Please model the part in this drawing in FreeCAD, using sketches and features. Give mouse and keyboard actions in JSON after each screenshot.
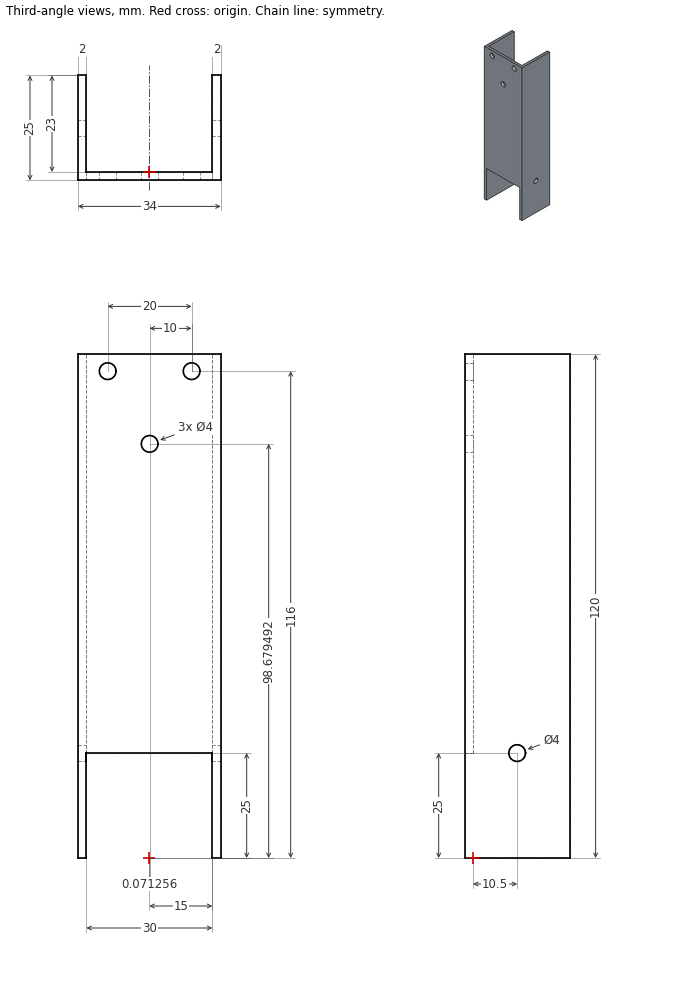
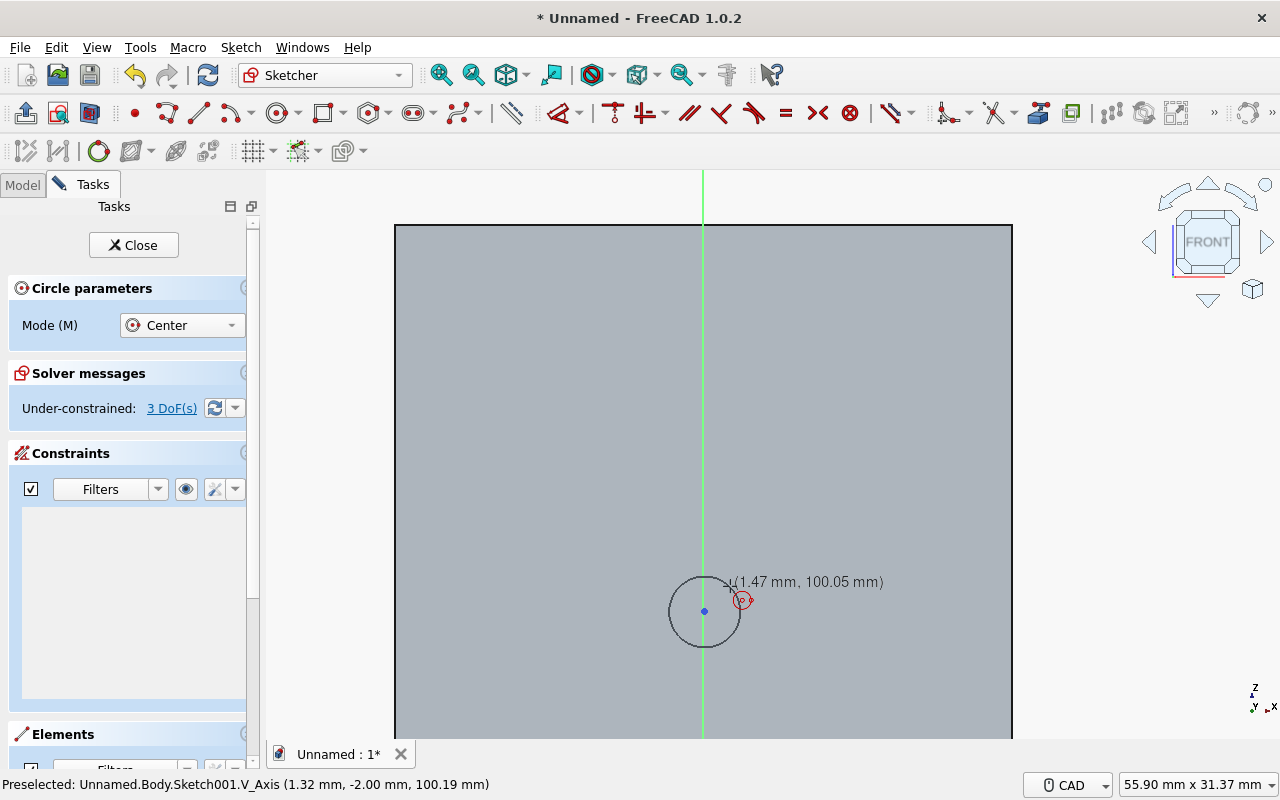
{"action": "left_click", "coordinate": [886, 298]}
{"action": "left_click", "coordinate": [912, 272]}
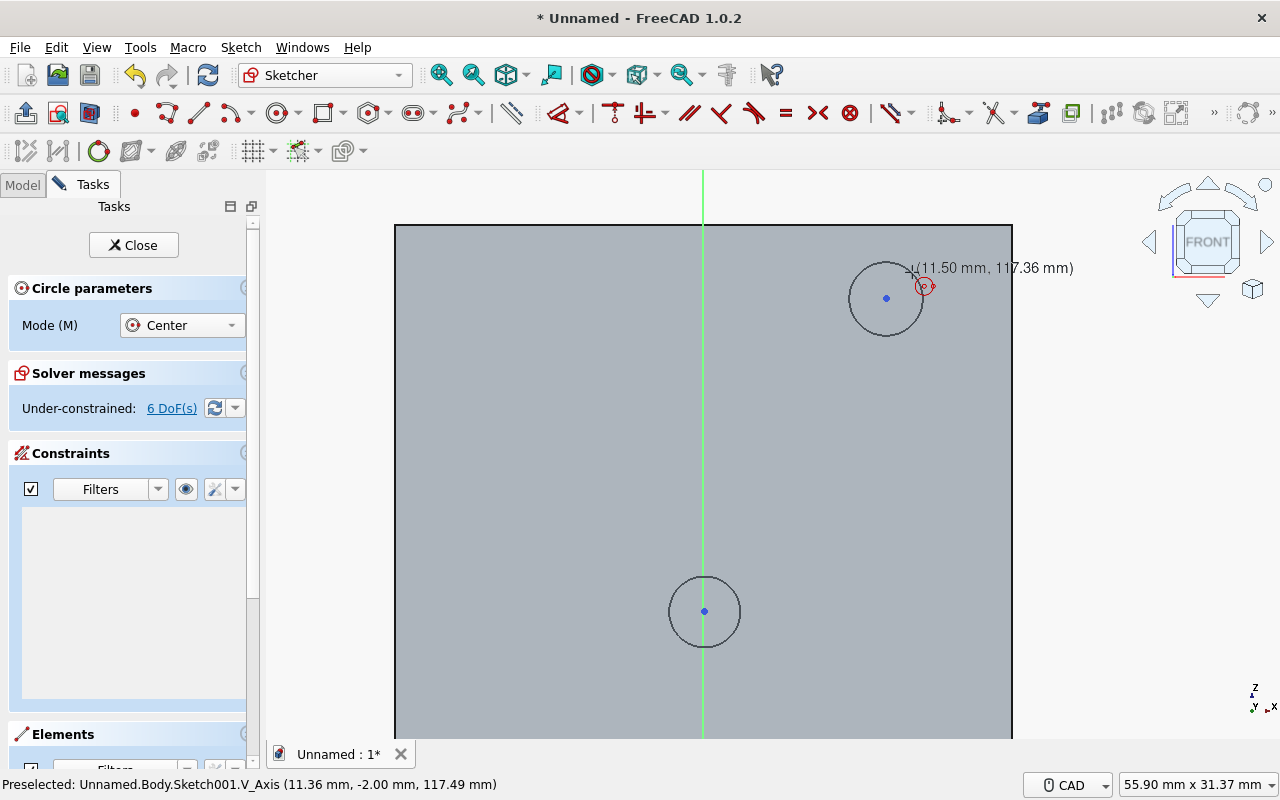
{"action": "left_click", "coordinate": [523, 298]}
{"action": "left_click", "coordinate": [549, 272]}
{"action": "key", "text": "Escape"}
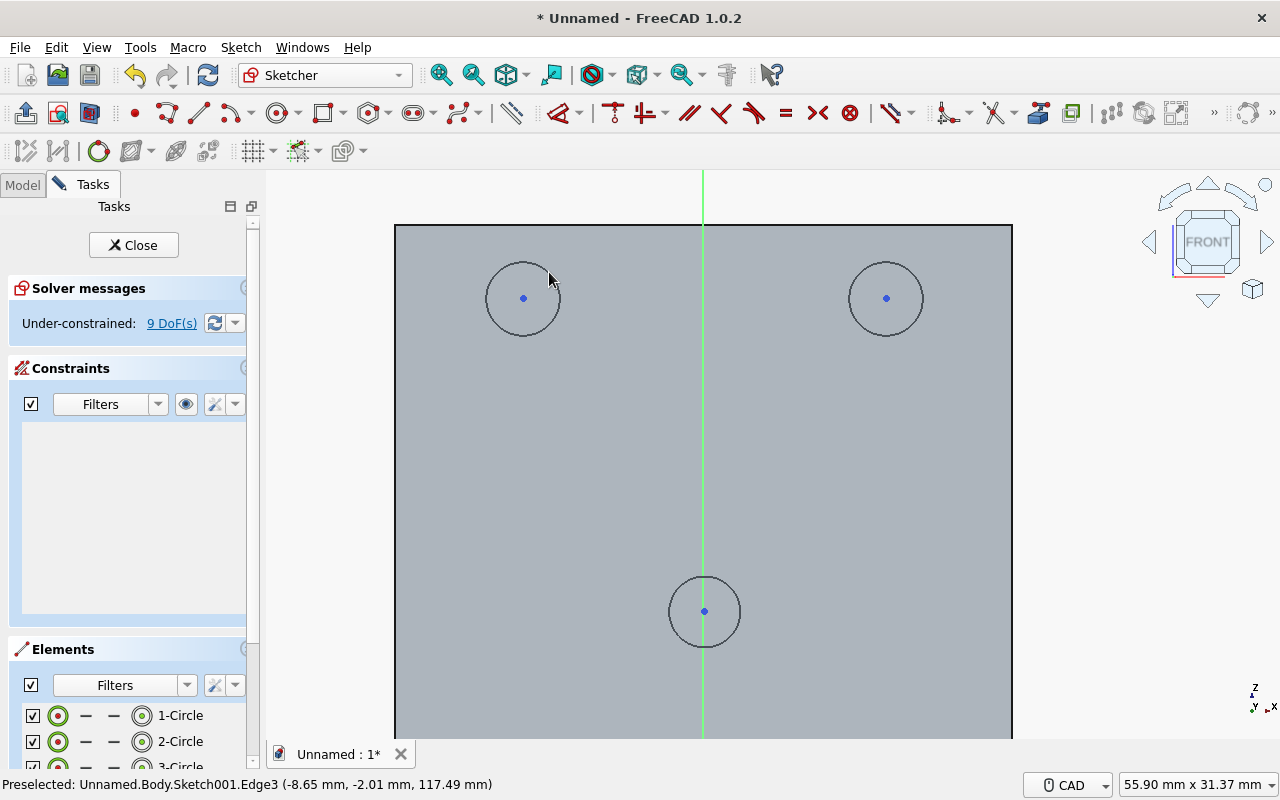
{"action": "left_click", "coordinate": [730, 587]}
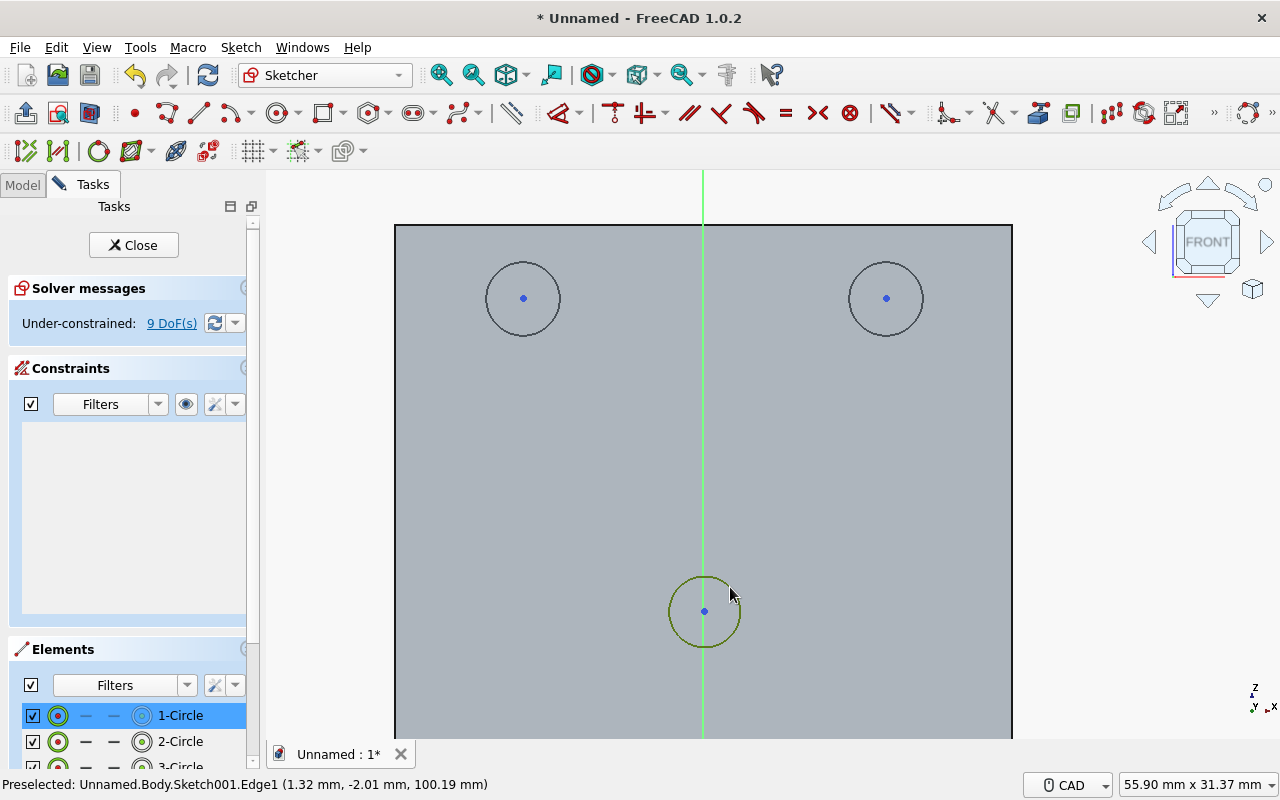
{"action": "left_click", "coordinate": [912, 273]}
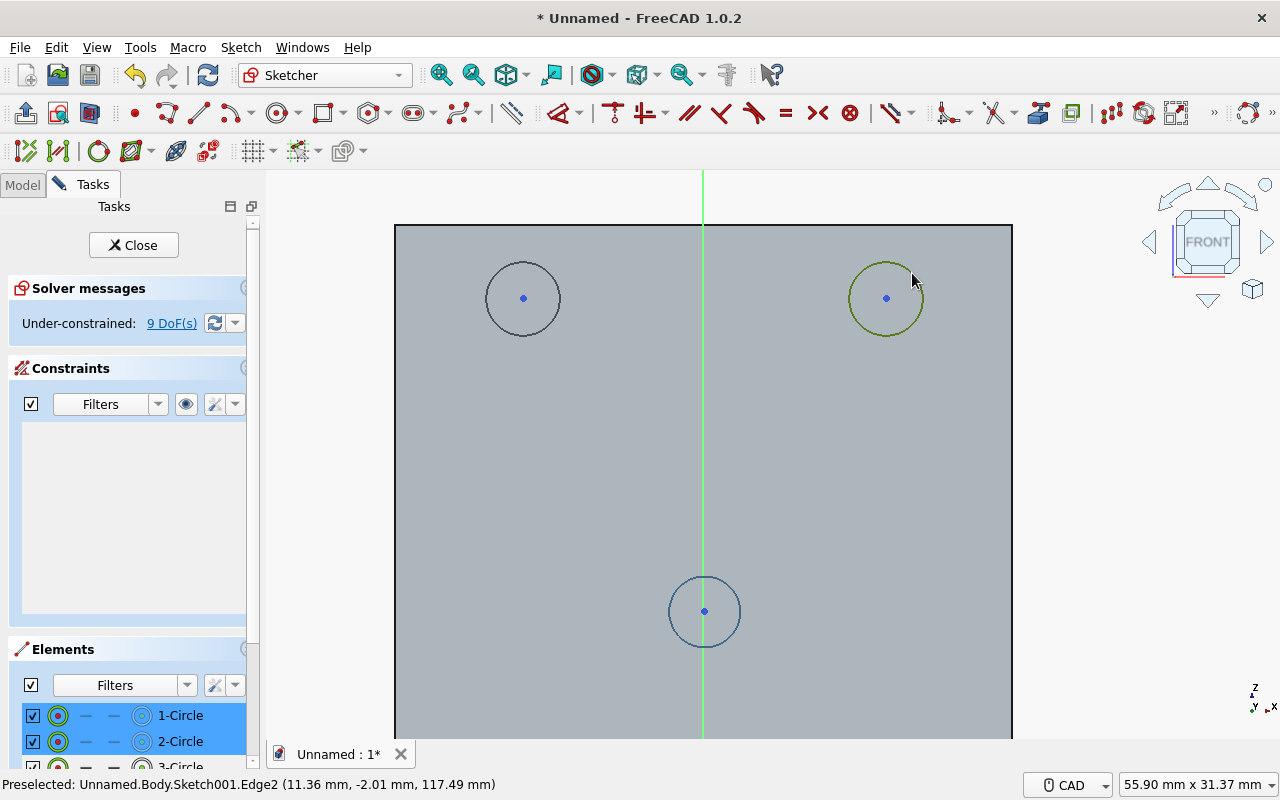
{"action": "left_click", "coordinate": [549, 273]}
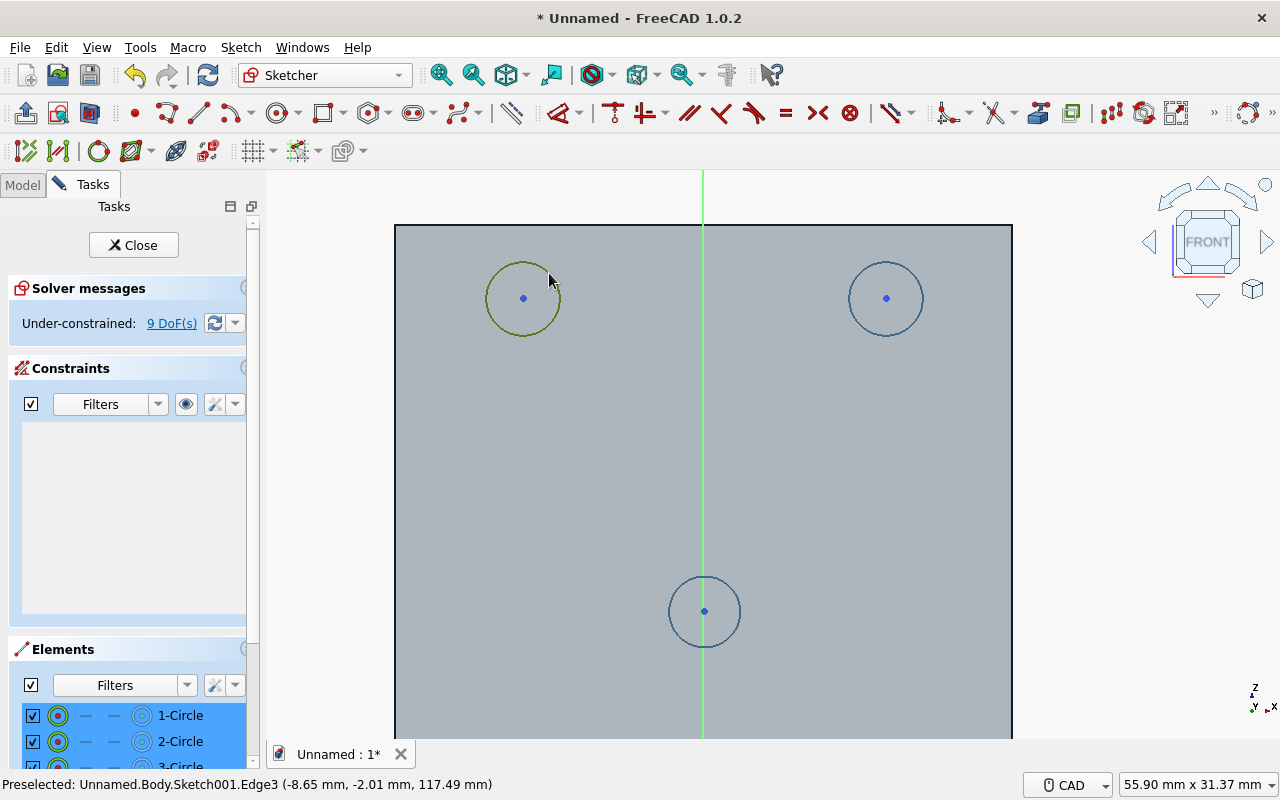
{"action": "left_click", "coordinate": [786, 114]}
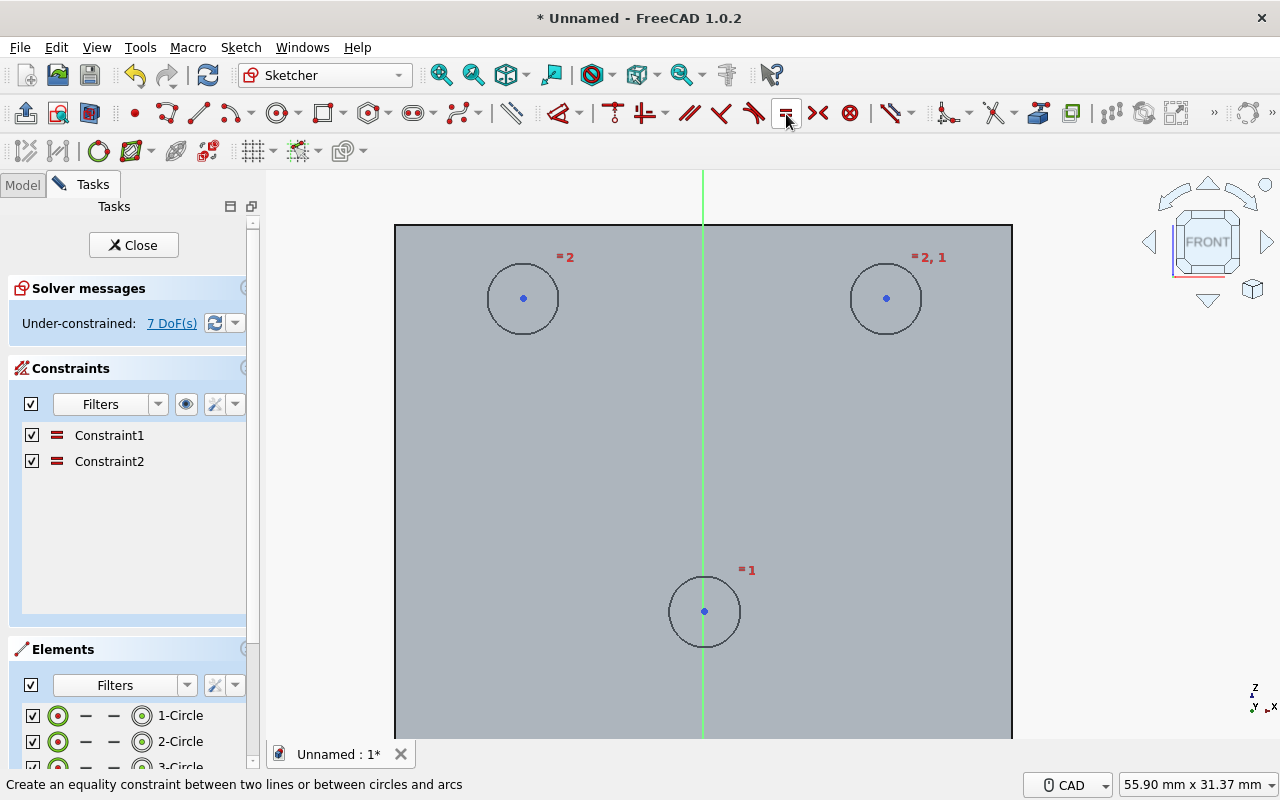
{"action": "left_click", "coordinate": [886, 299]}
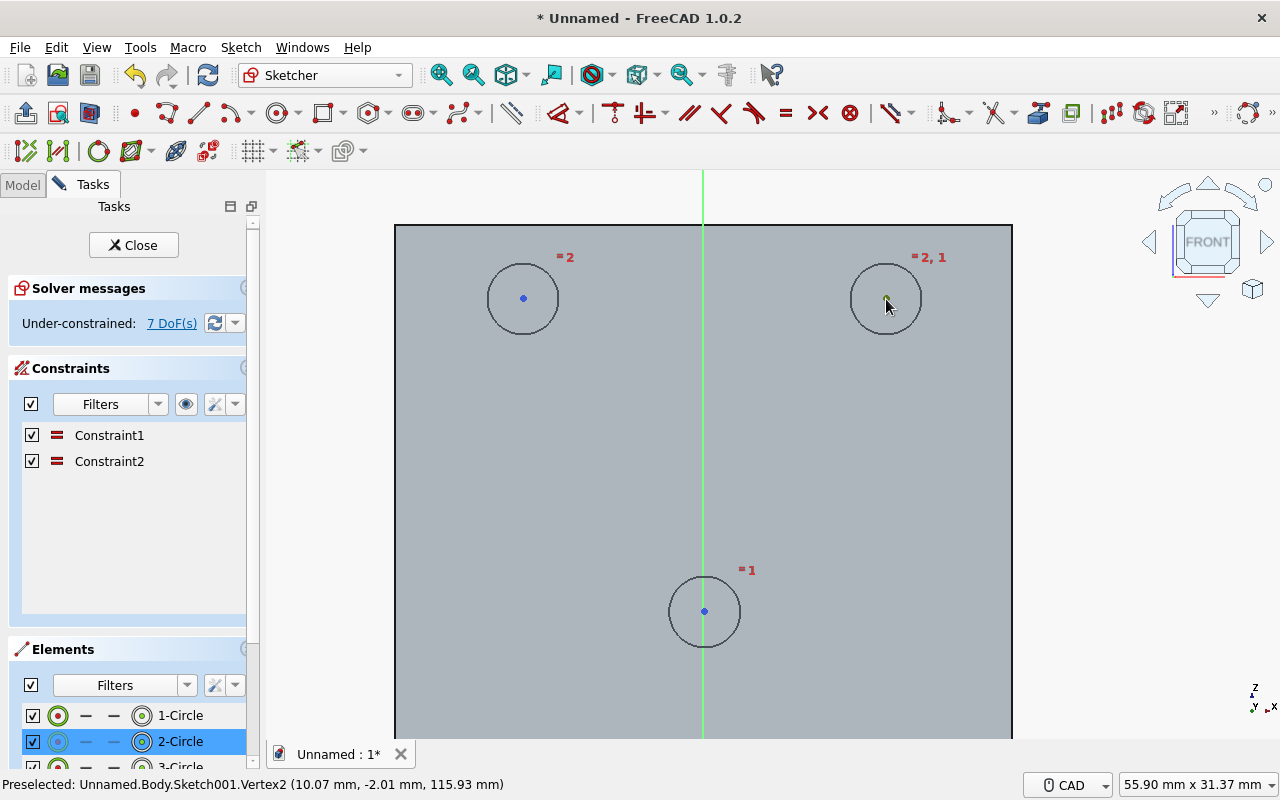
{"action": "left_click", "coordinate": [523, 299]}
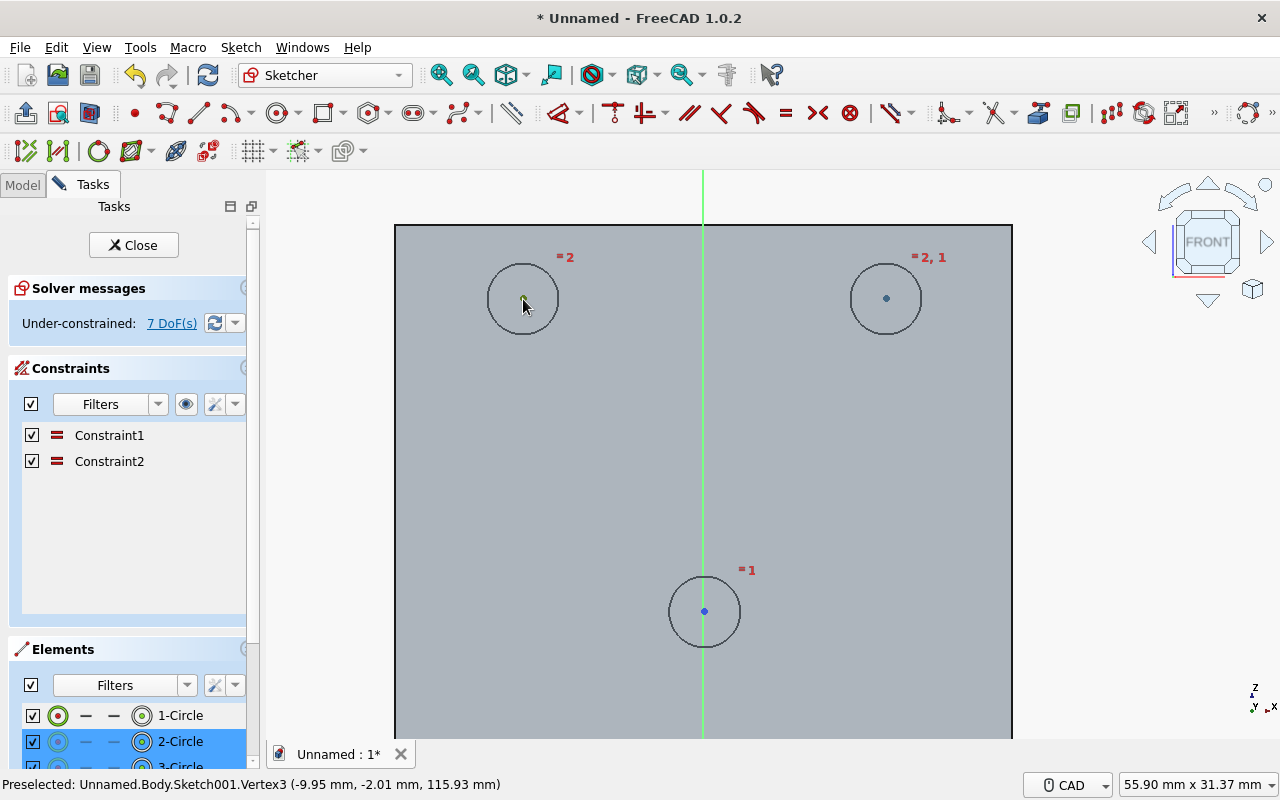
{"action": "left_click", "coordinate": [668, 114]}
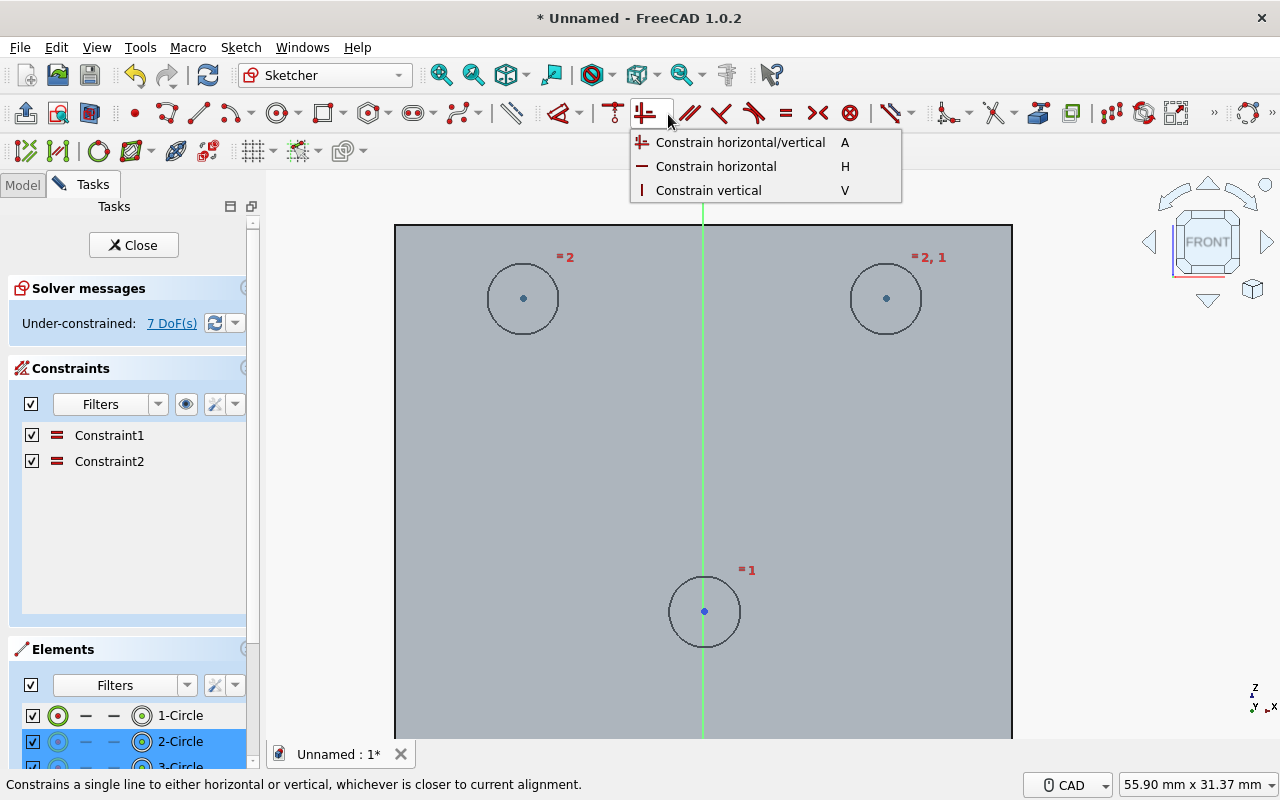
{"action": "left_click", "coordinate": [766, 166]}